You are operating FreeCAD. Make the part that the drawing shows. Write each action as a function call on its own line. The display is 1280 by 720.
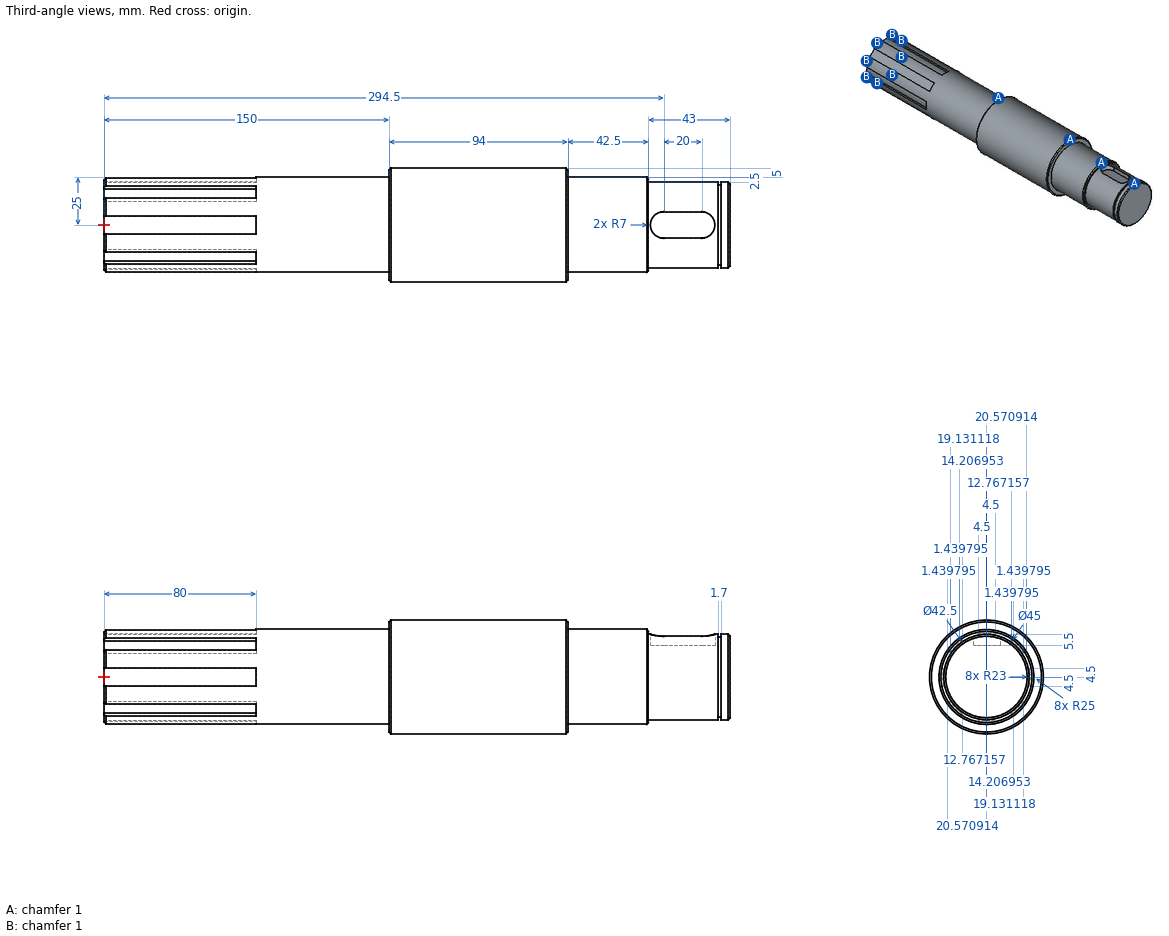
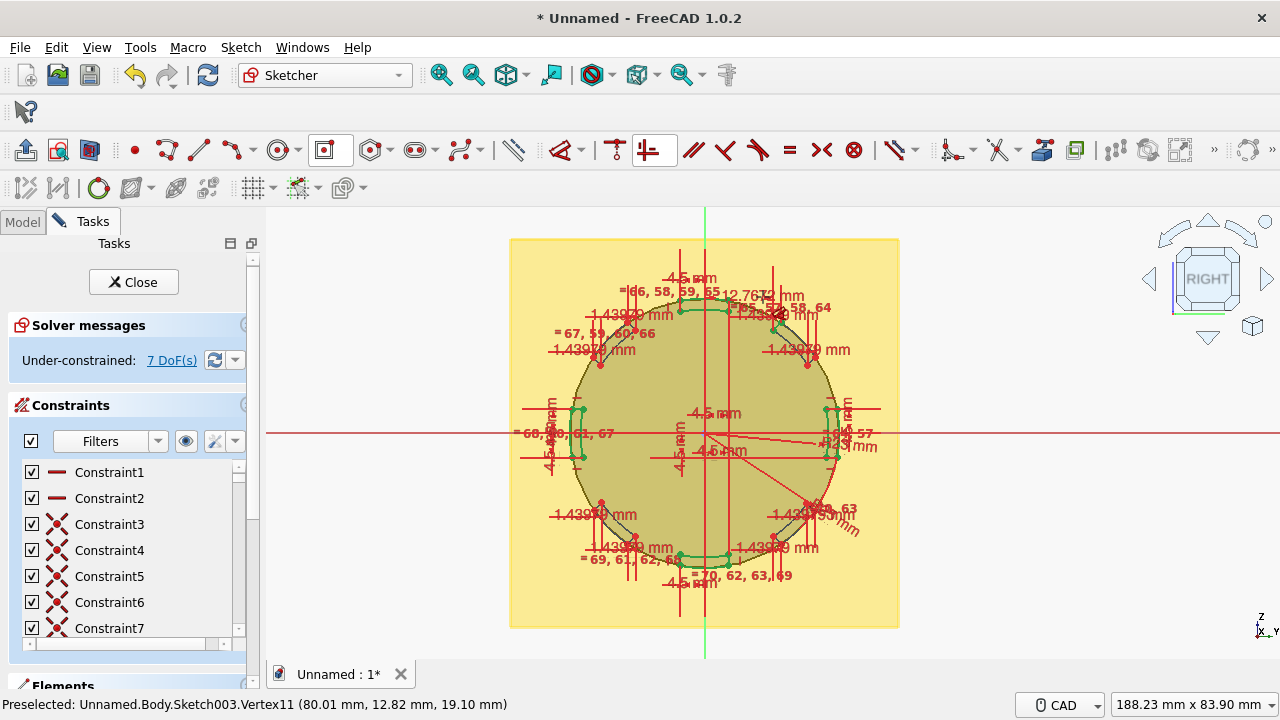
click(816, 357)
click(799, 467)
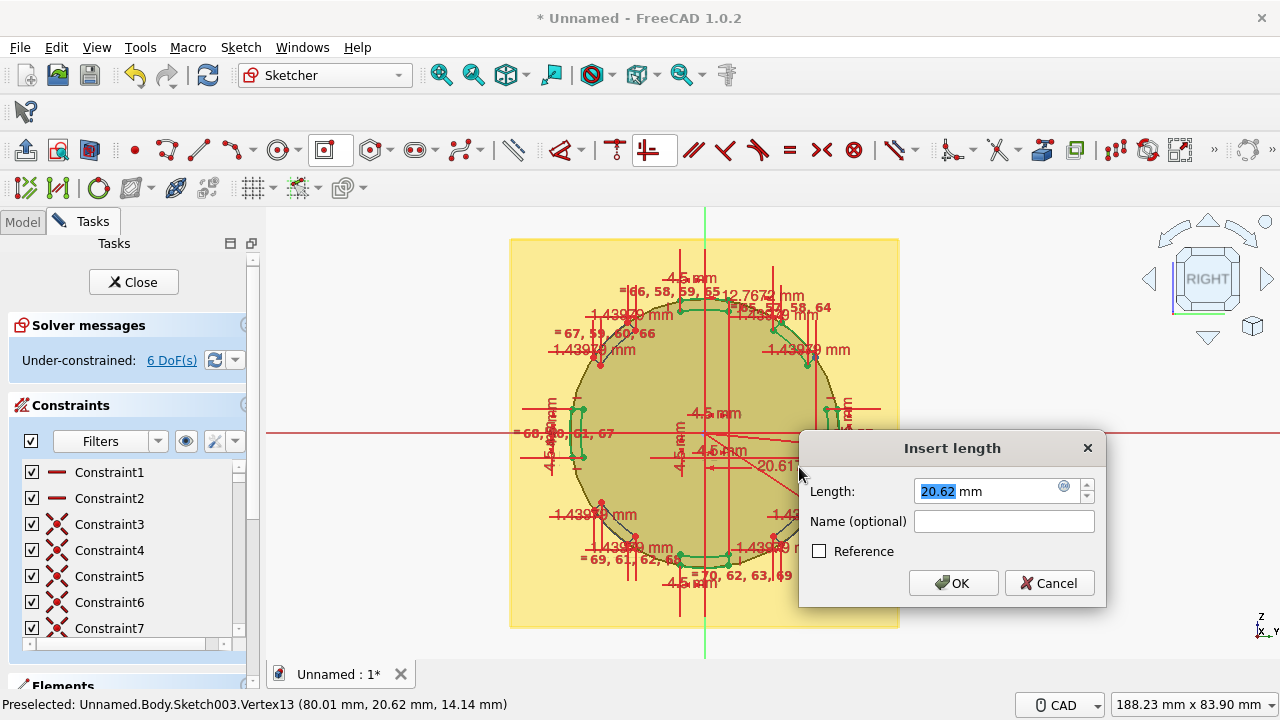
text(20.570914)
key(Return)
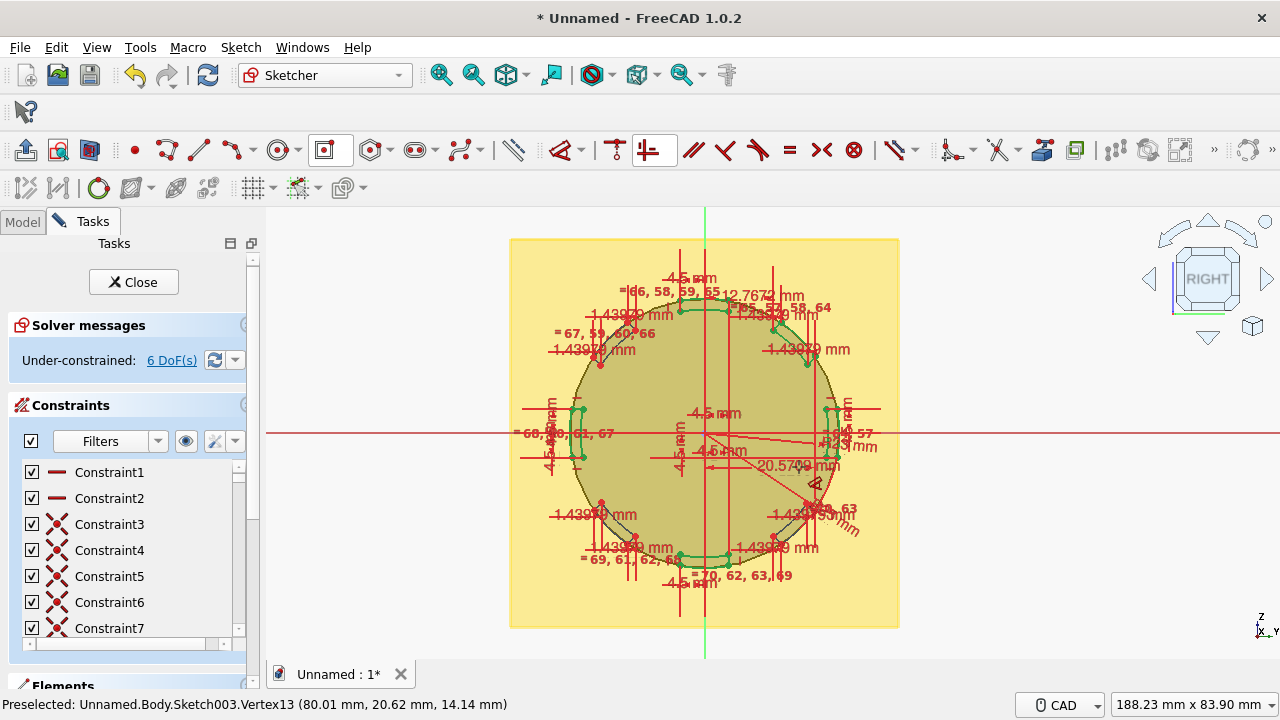
click(601, 365)
click(629, 467)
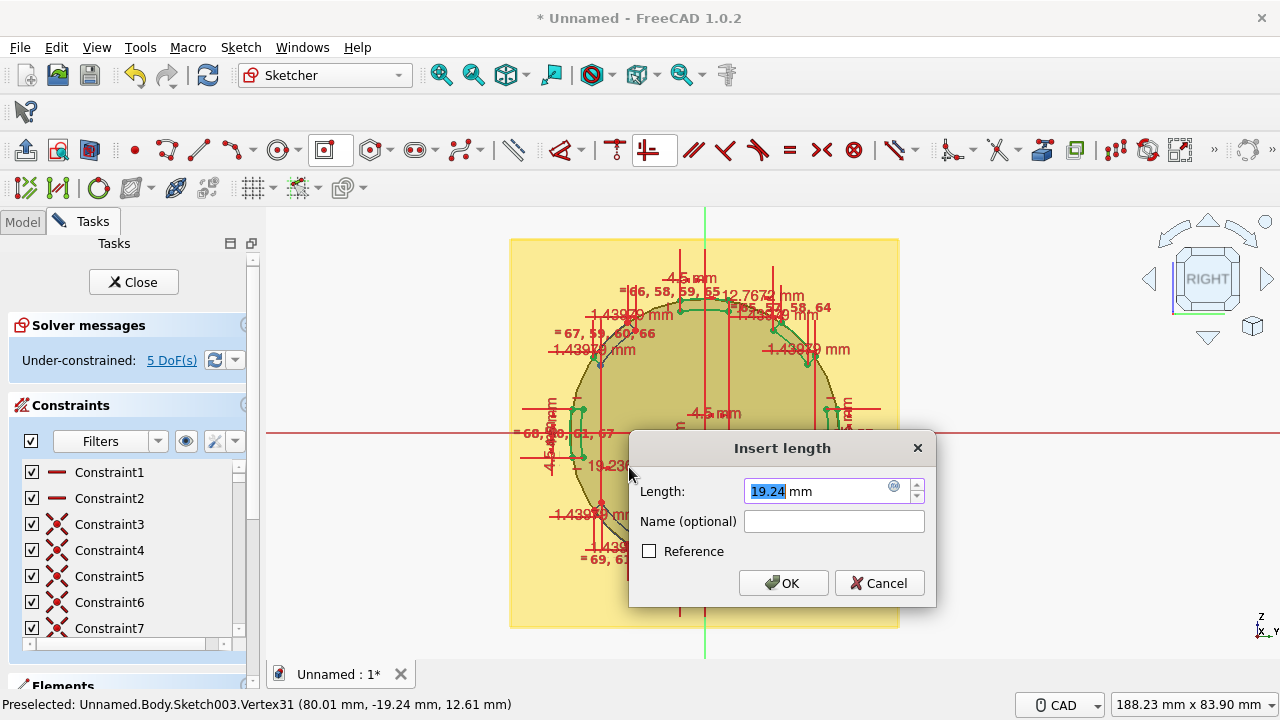
text(19.131118)
key(Return)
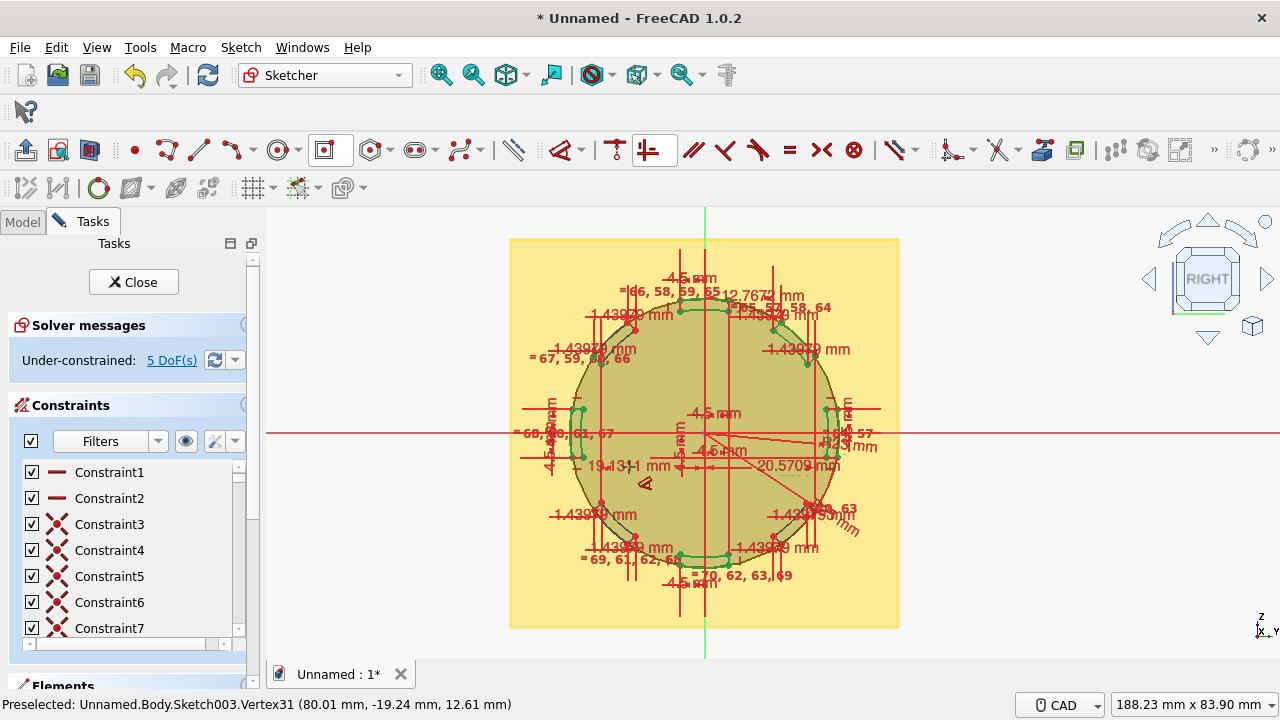
click(628, 323)
click(666, 491)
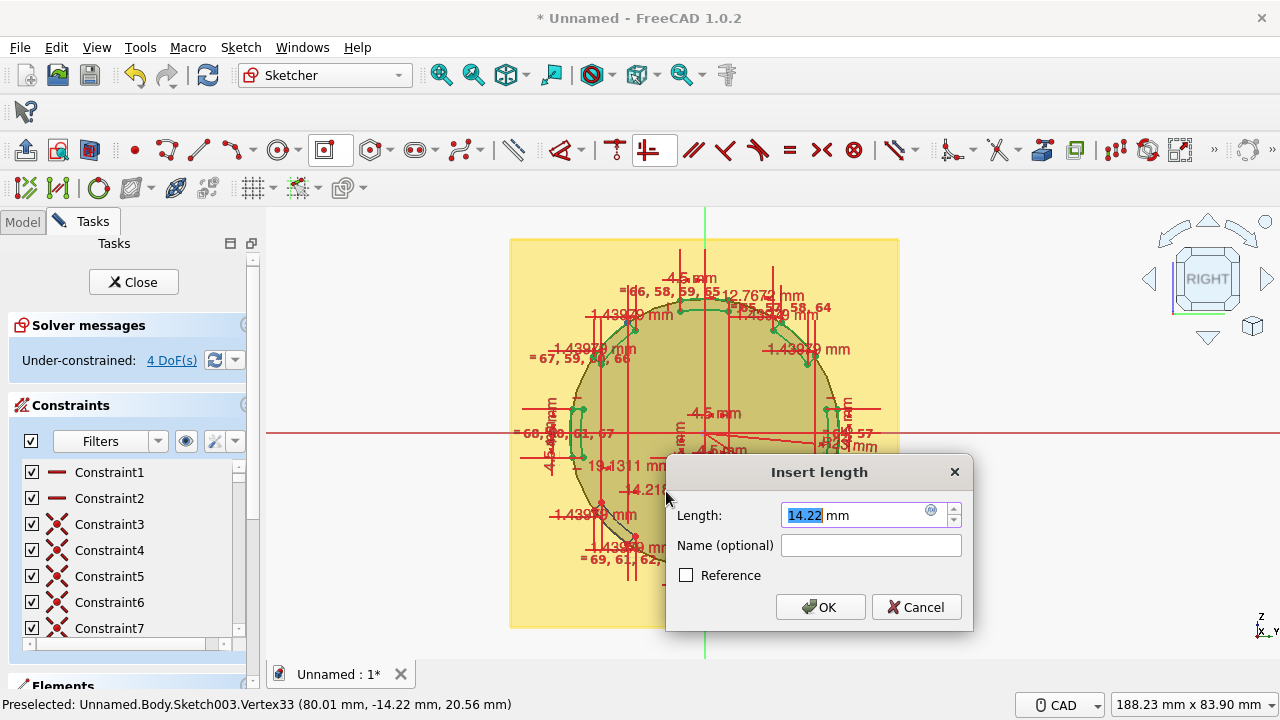
text(14.206953)
key(Return)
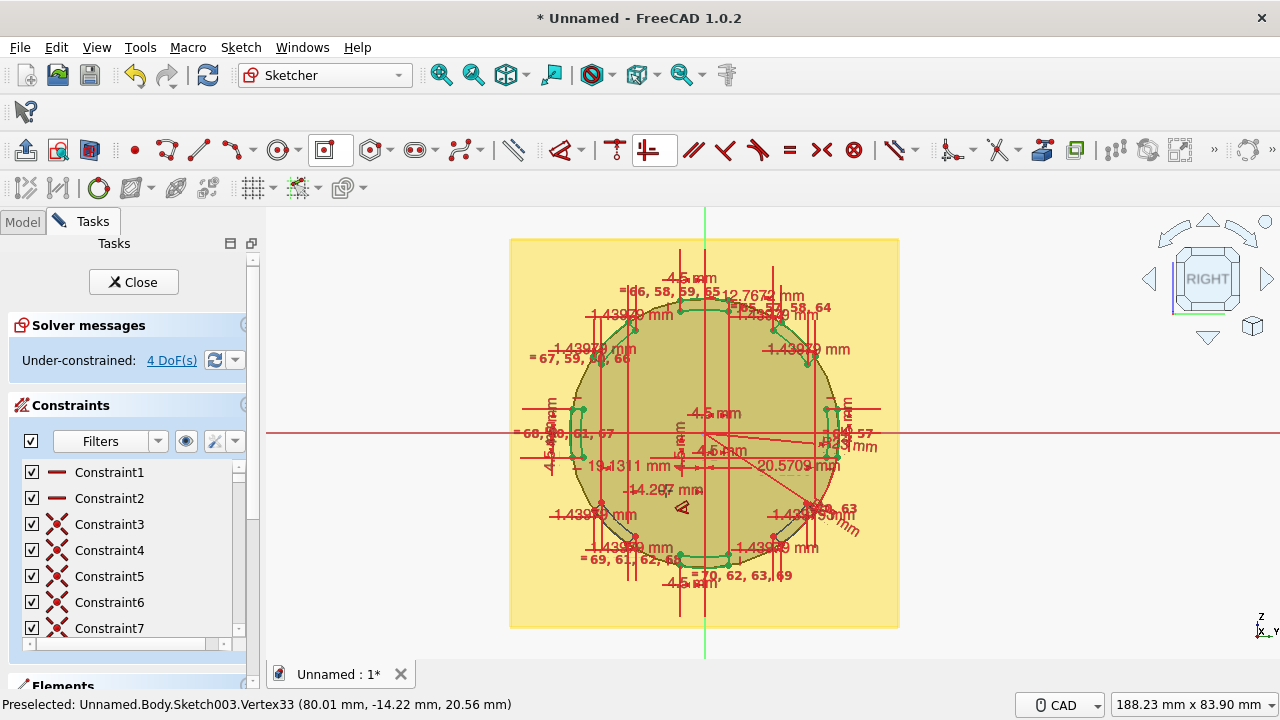
click(636, 536)
click(646, 399)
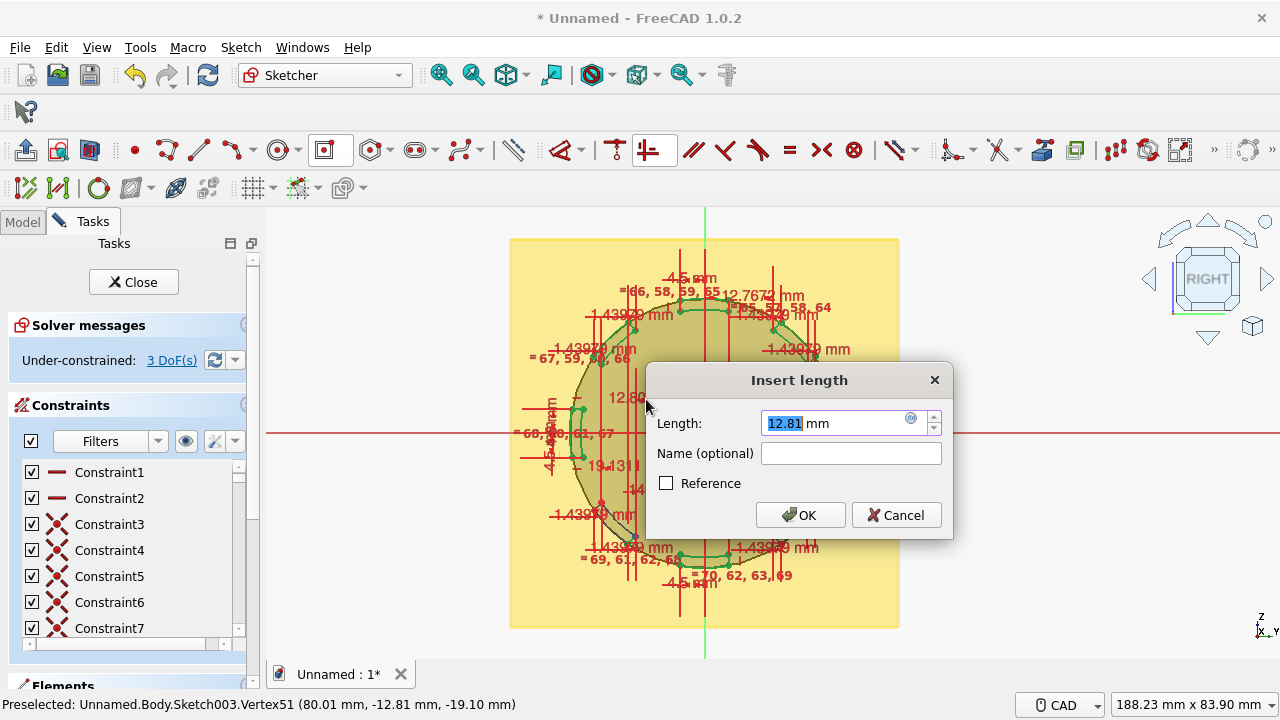
text(12.767157)
key(Return)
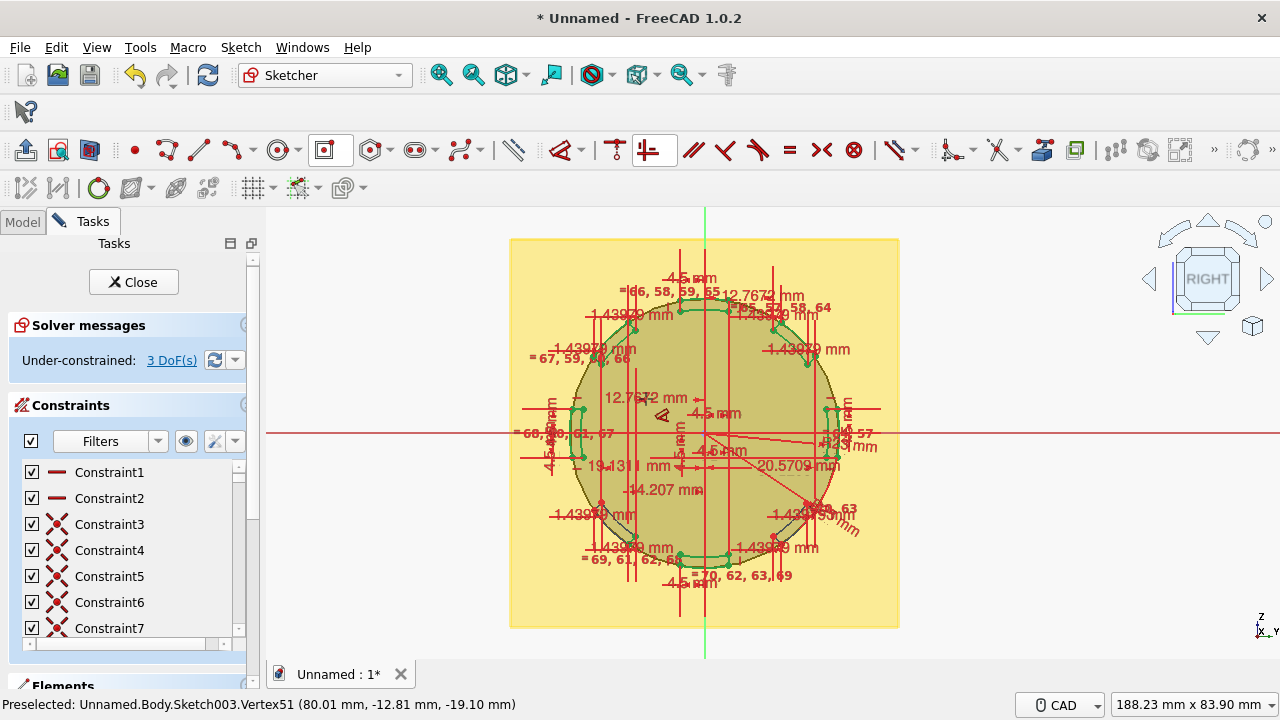
click(594, 511)
click(649, 375)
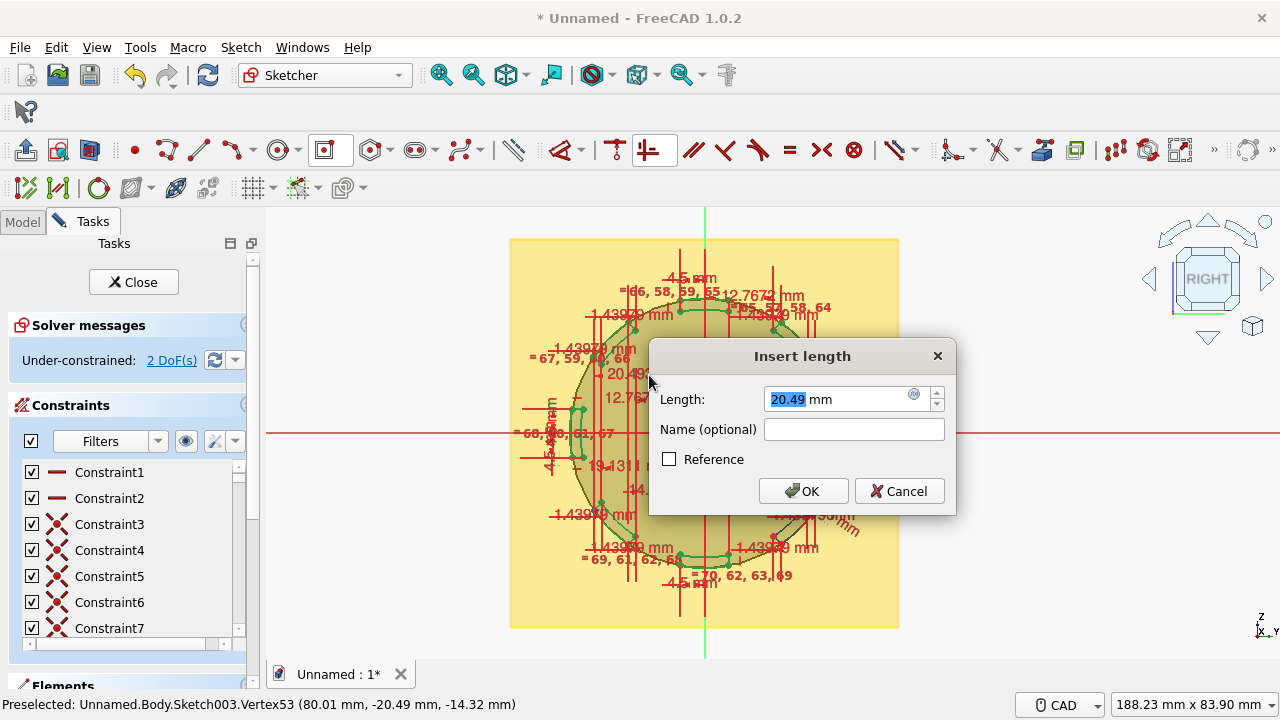
text(20.570914)
key(Return)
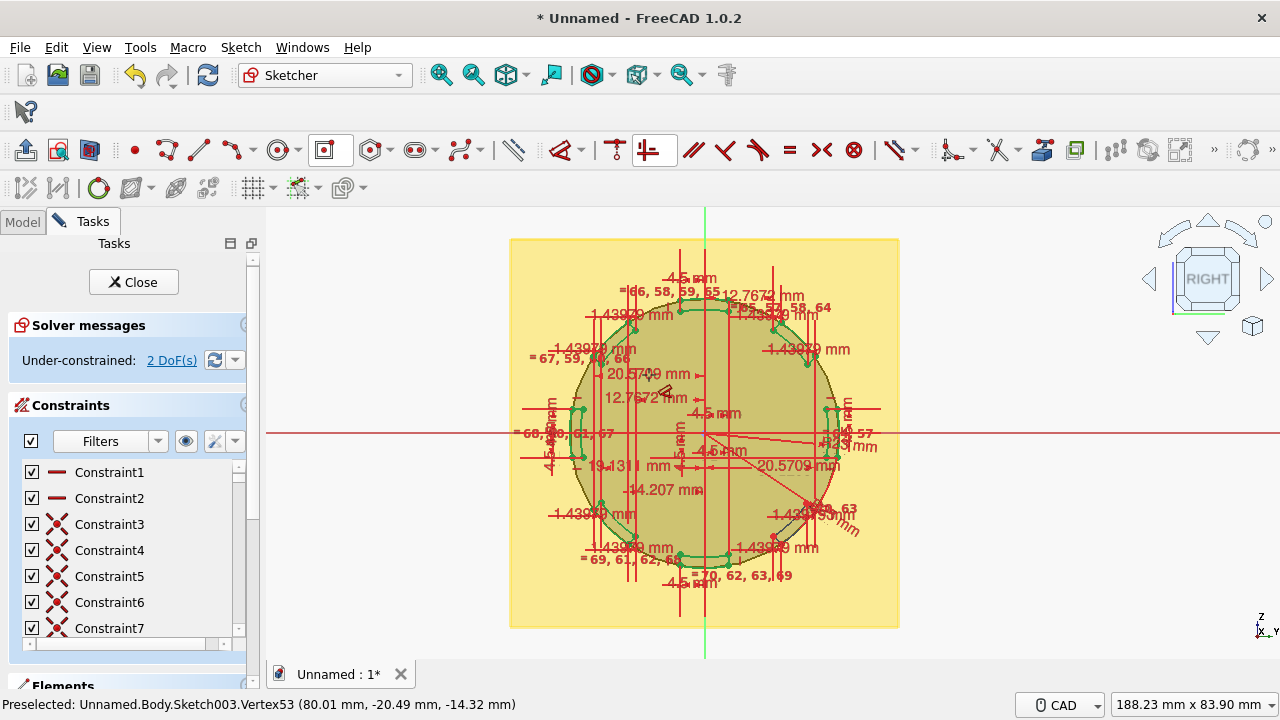
click(807, 503)
click(791, 399)